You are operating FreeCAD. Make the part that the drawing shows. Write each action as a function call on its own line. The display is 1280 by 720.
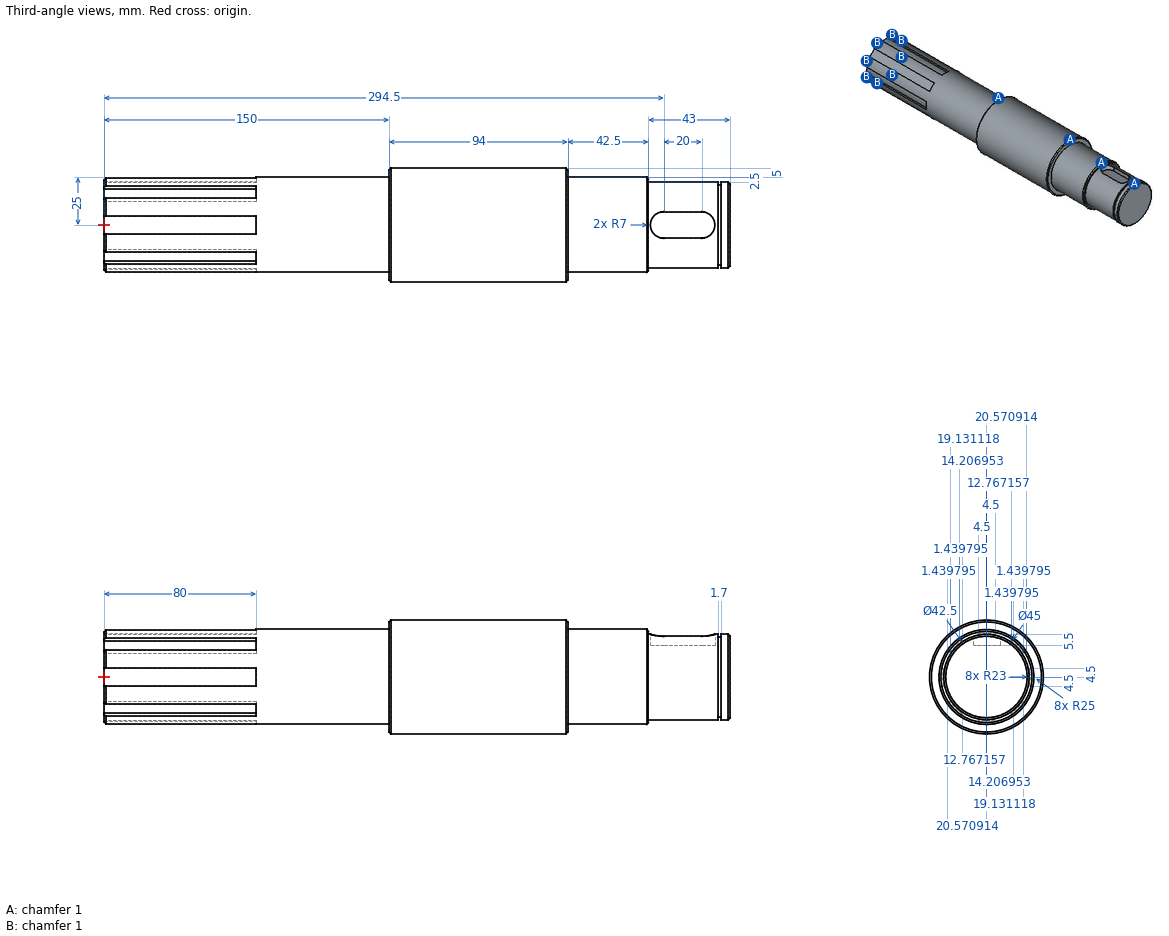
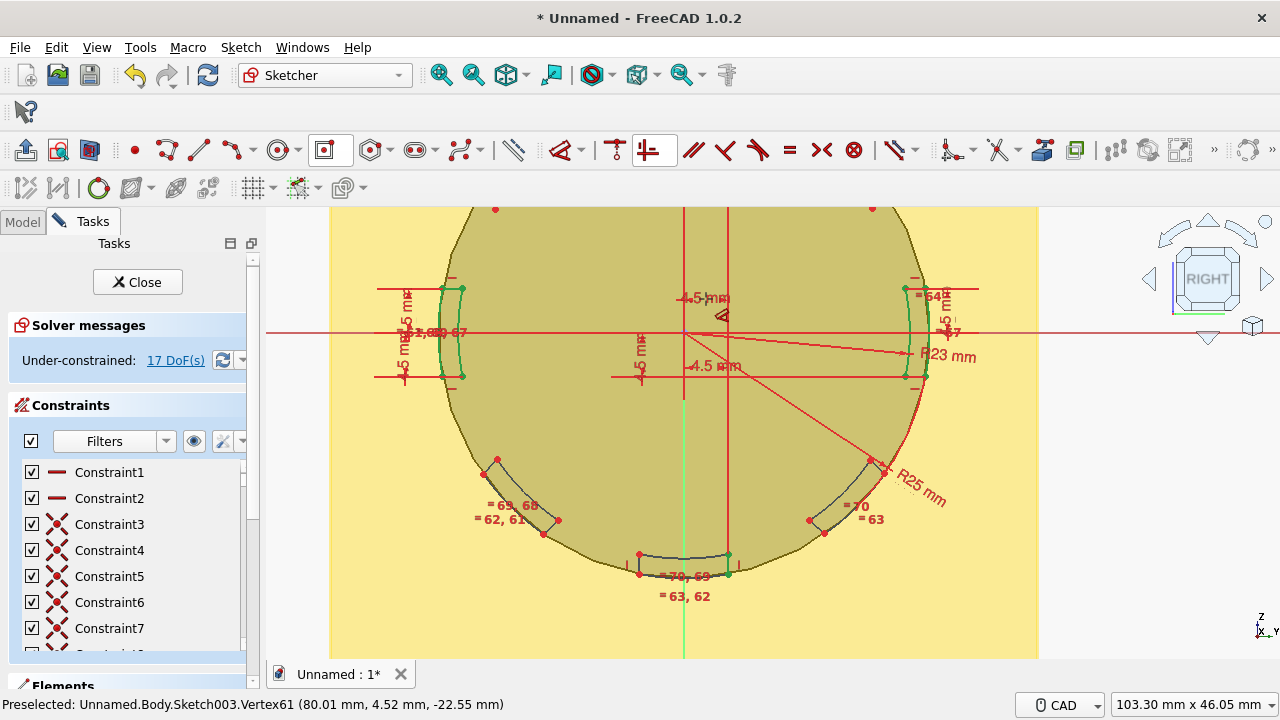
click(639, 574)
click(662, 608)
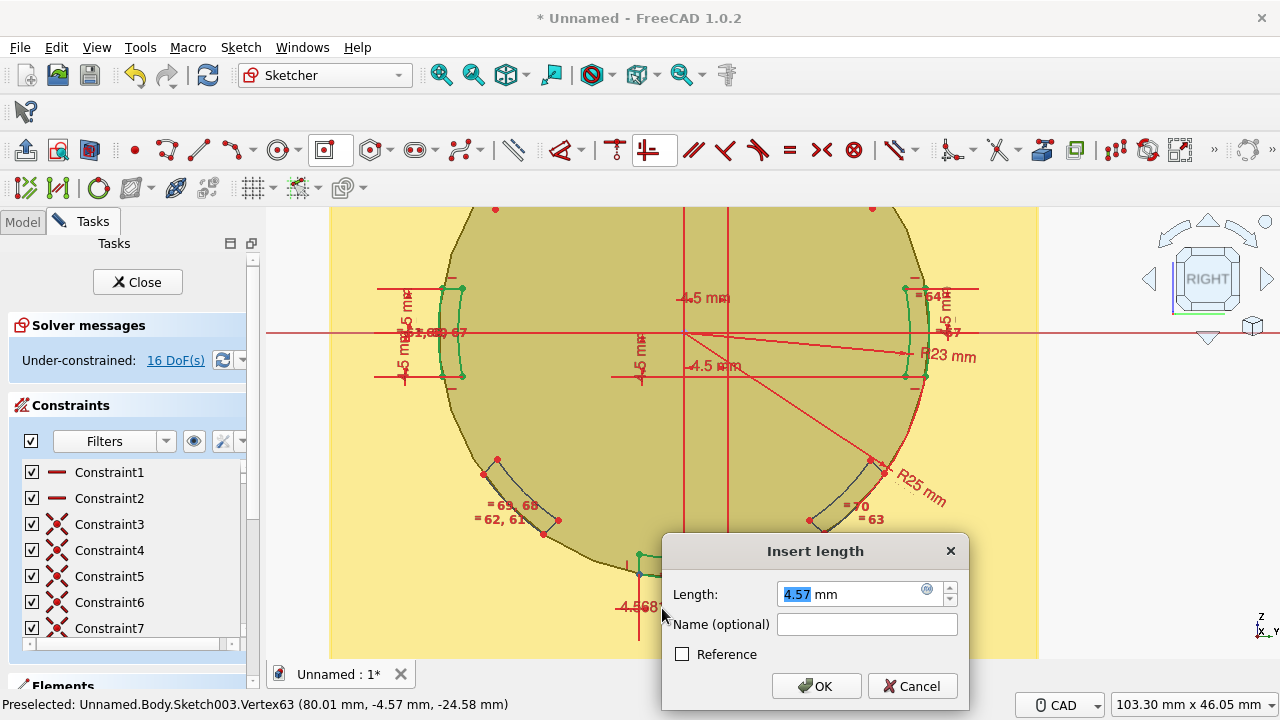
text(4.5)
key(Return)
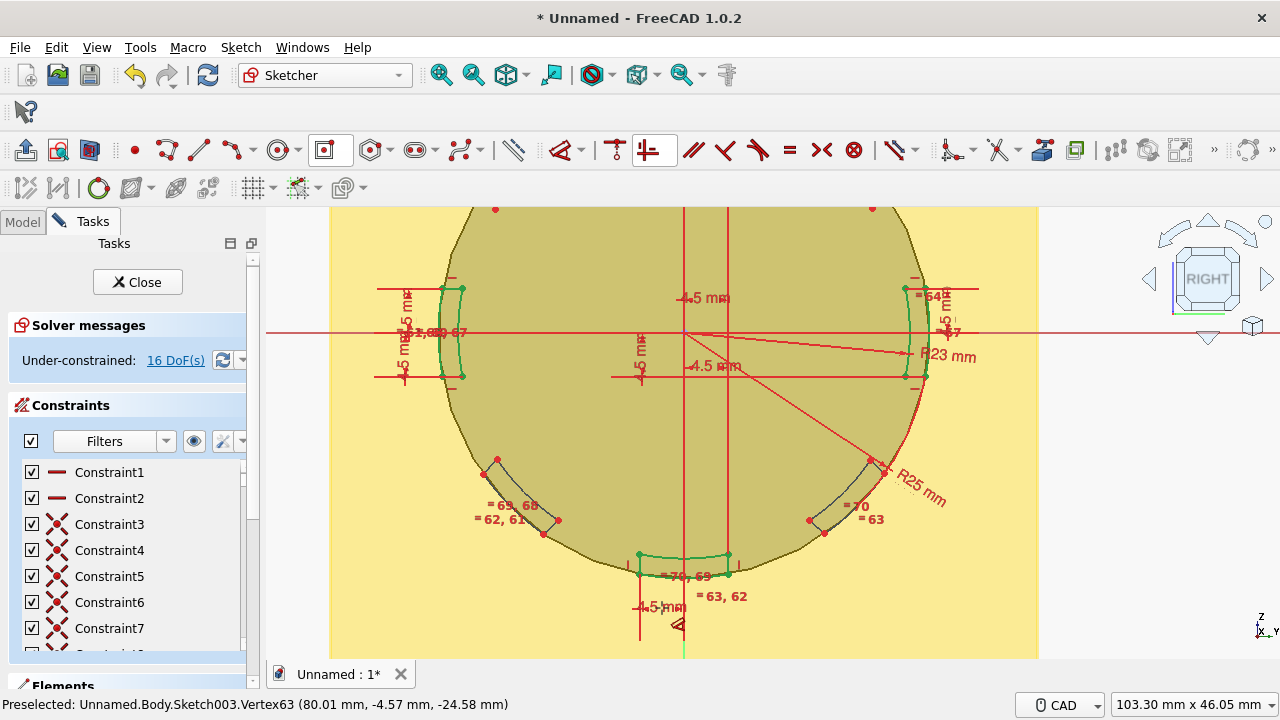
scroll(729, 555, down, 3)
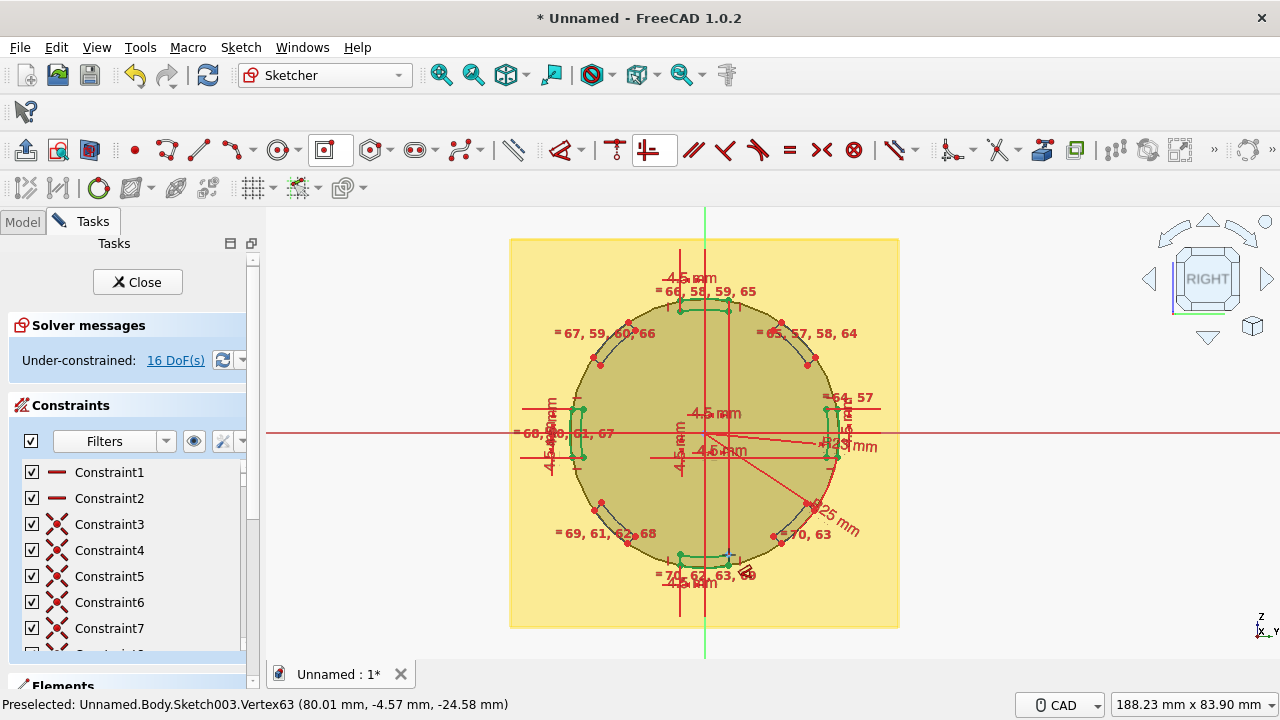
scroll(777, 326, up, 9)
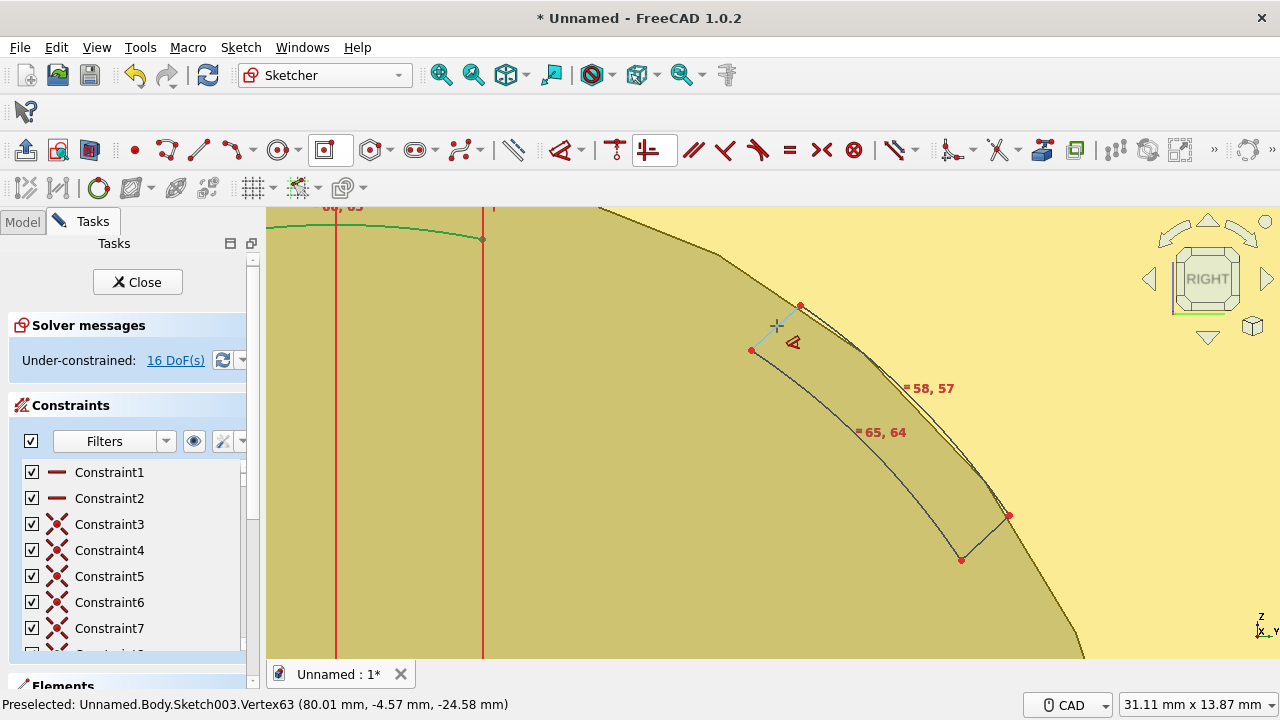
click(776, 328)
click(776, 271)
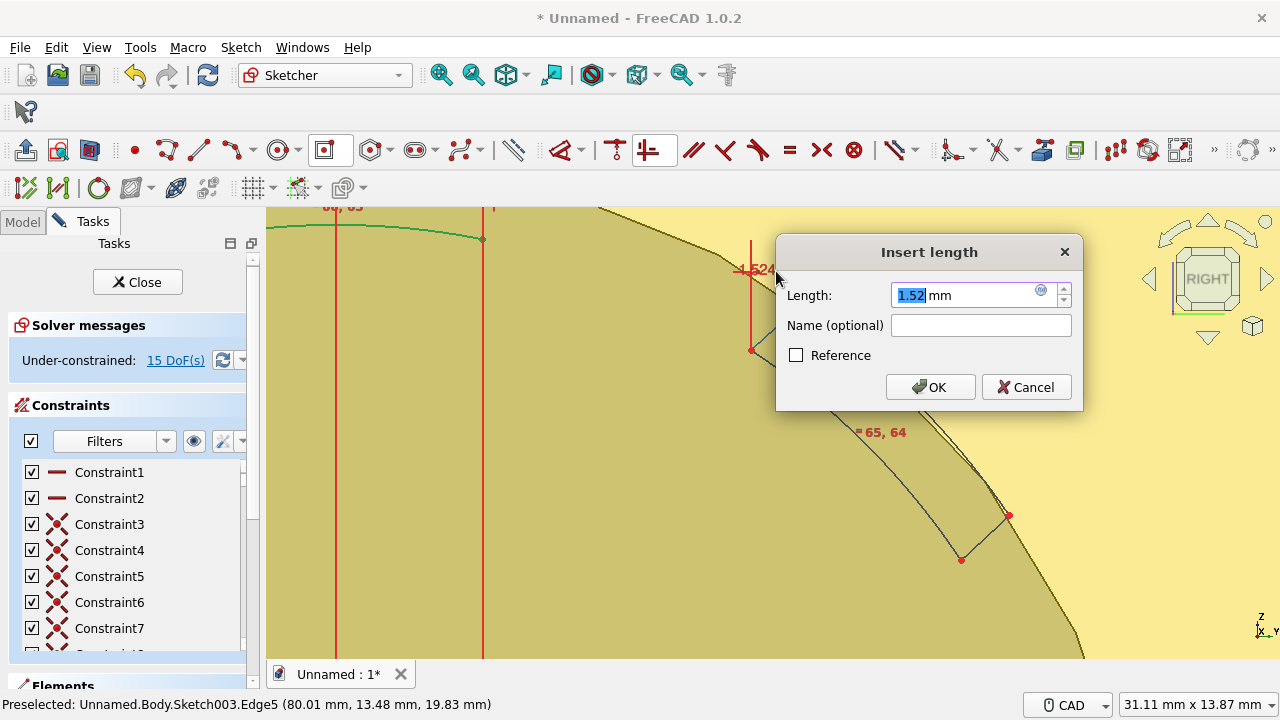
text(1.439795)
key(Return)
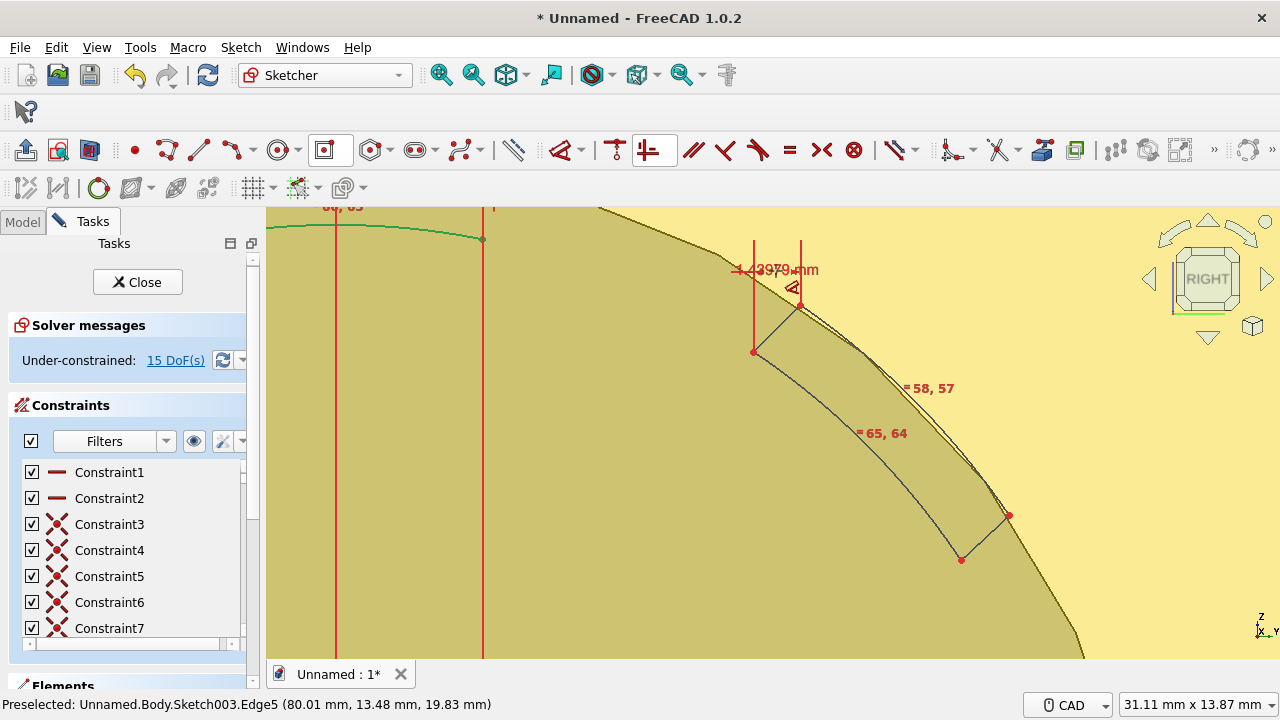
click(995, 529)
click(968, 482)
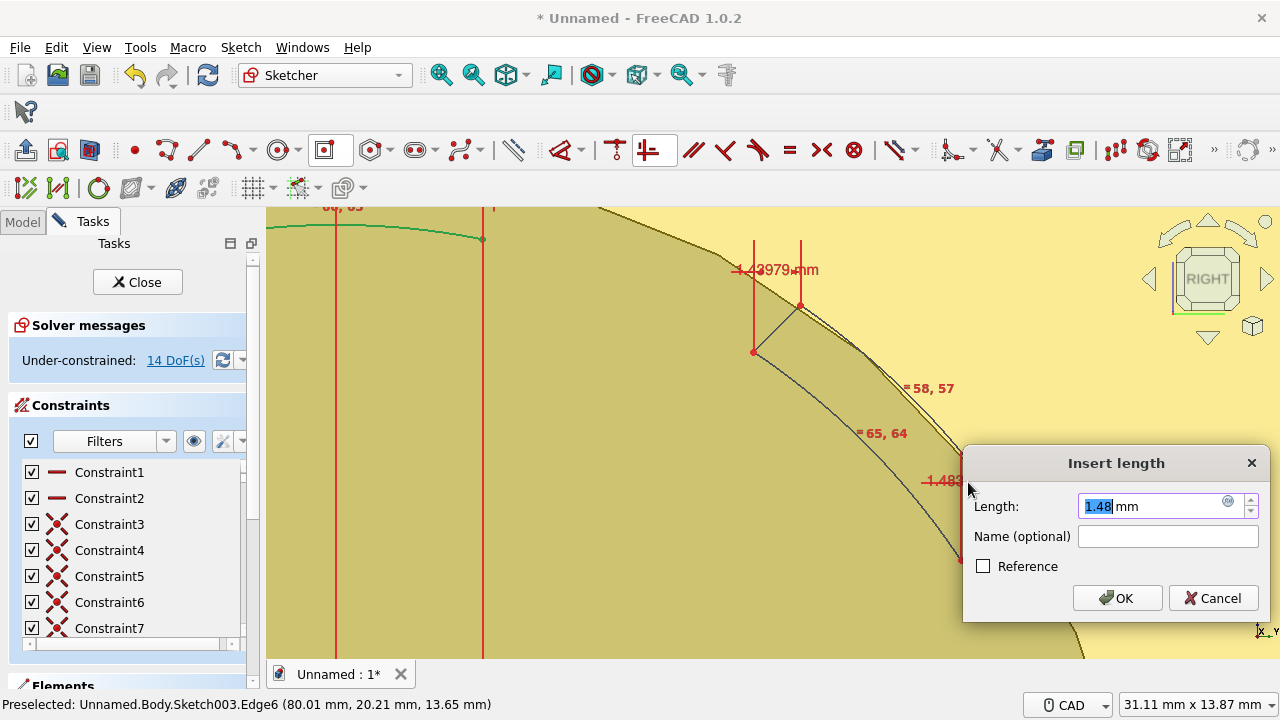
text(1.439795)
key(Return)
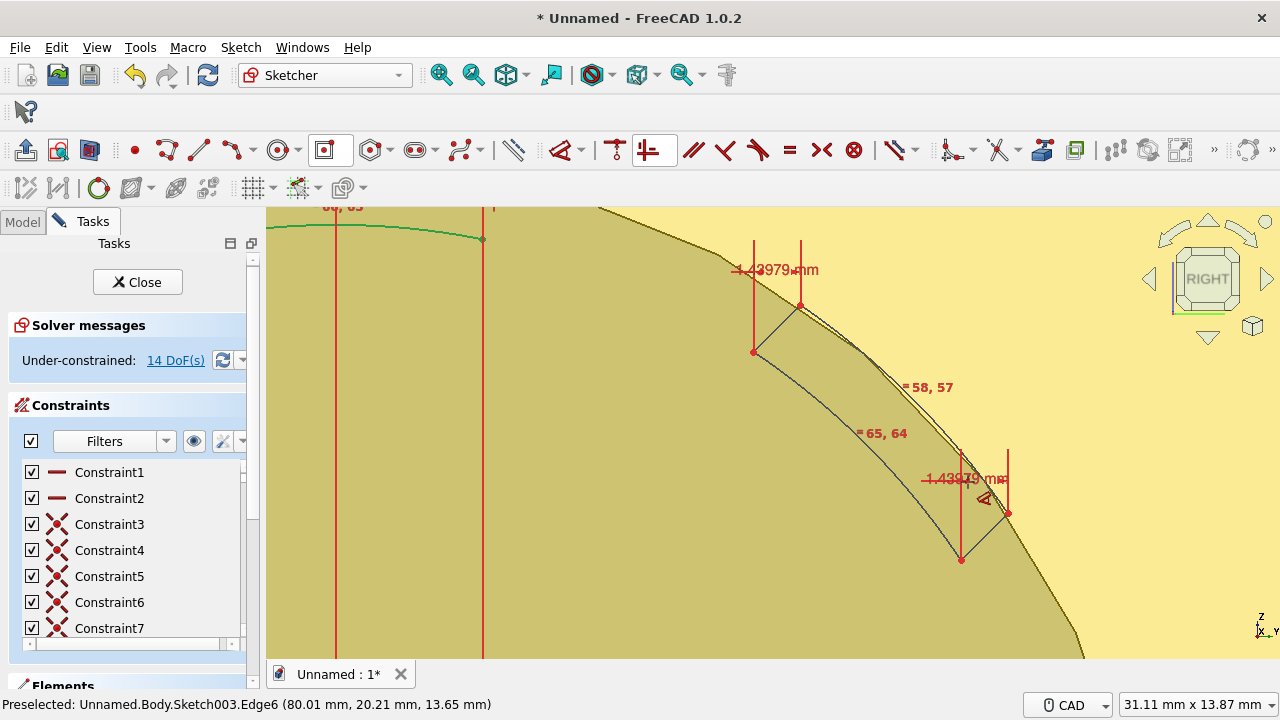
scroll(777, 326, down, 9)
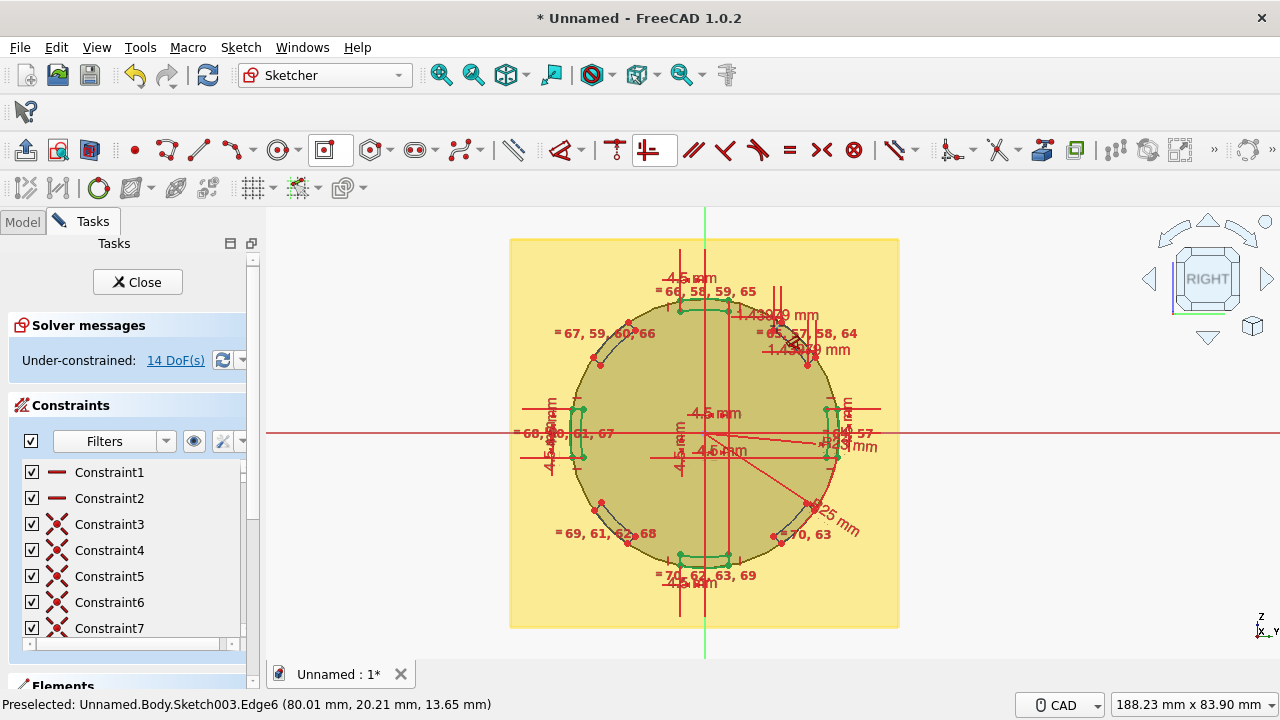
scroll(599, 363, up, 9)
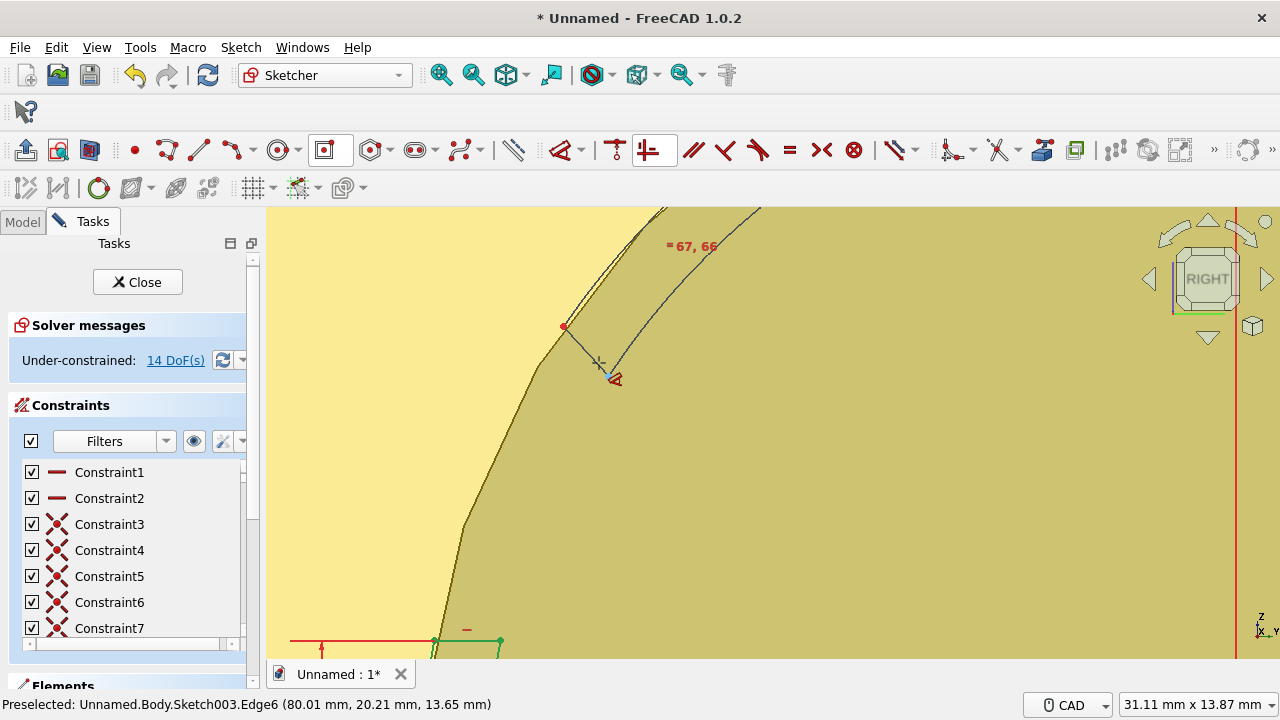
click(595, 361)
click(570, 293)